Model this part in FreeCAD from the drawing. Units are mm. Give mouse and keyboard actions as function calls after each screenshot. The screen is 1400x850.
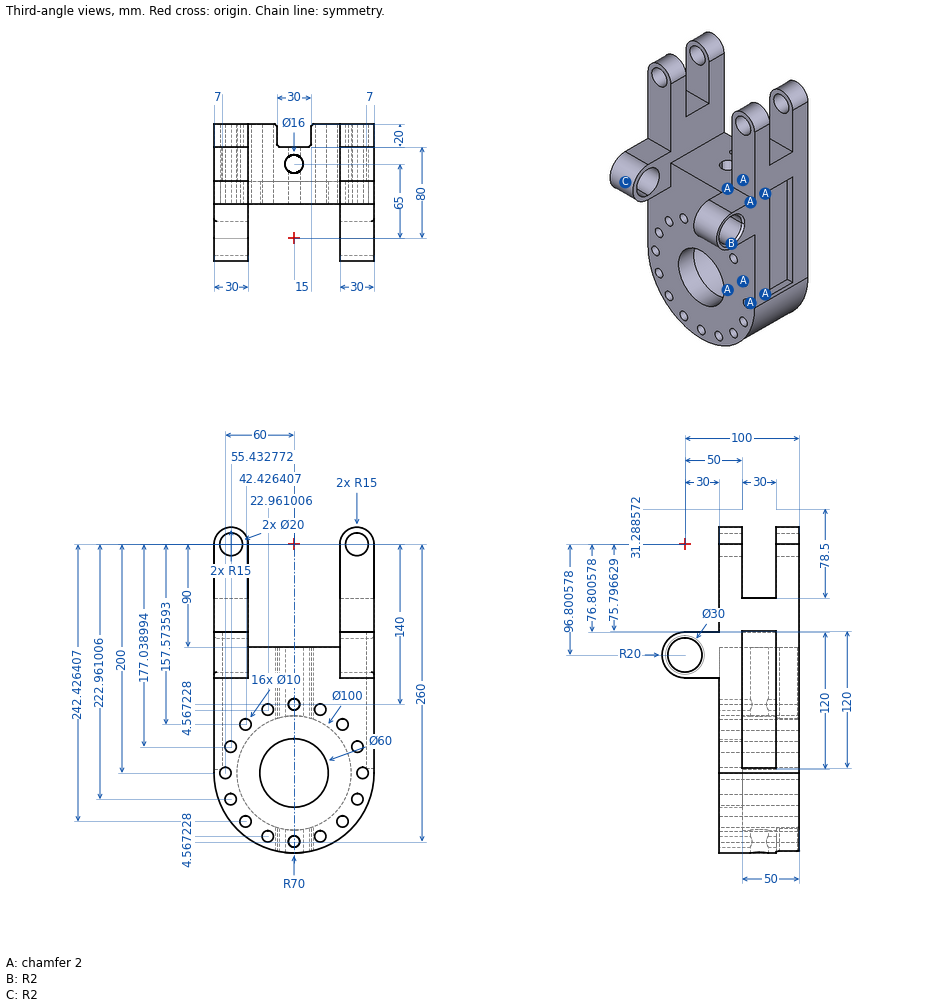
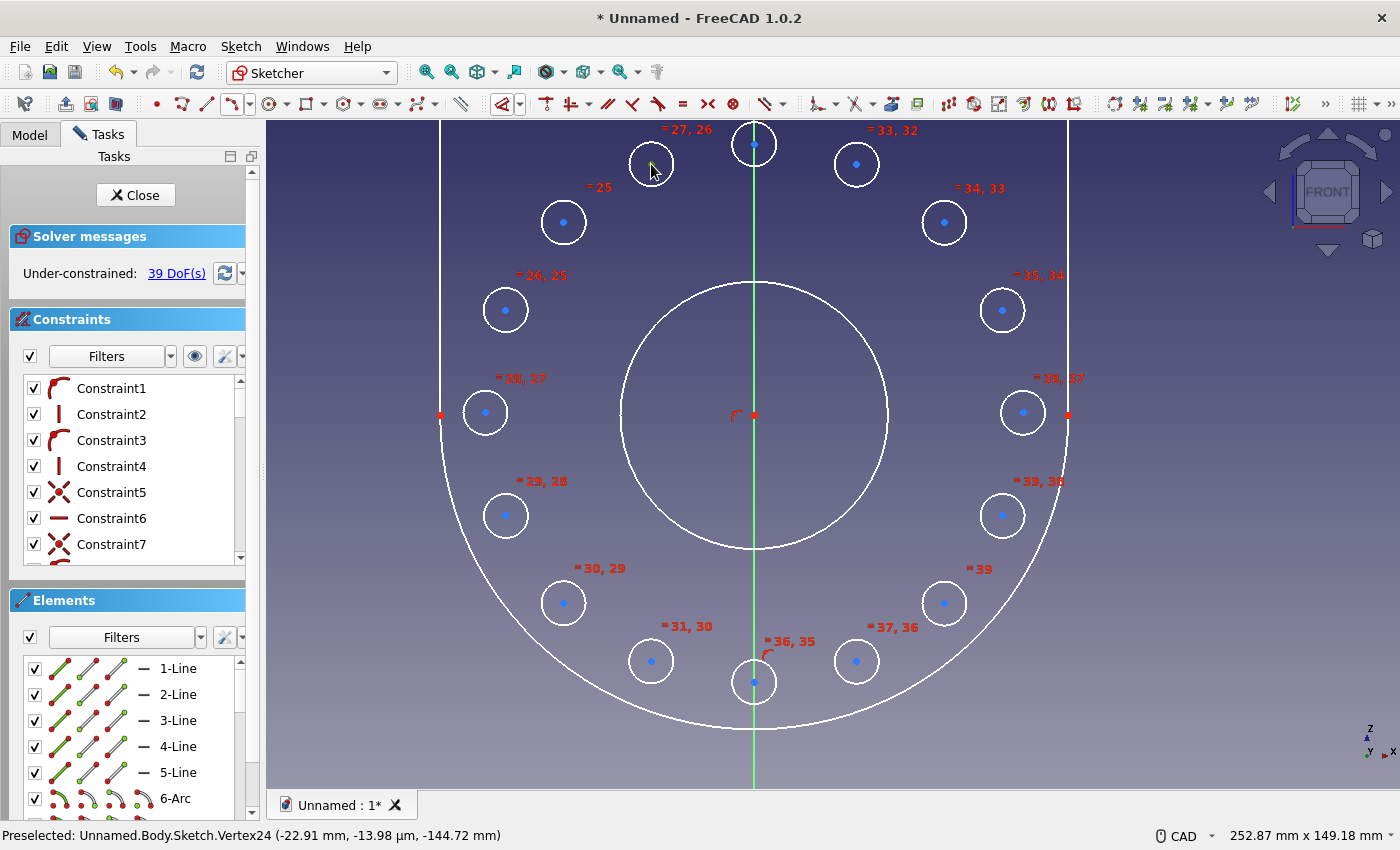
click(857, 165)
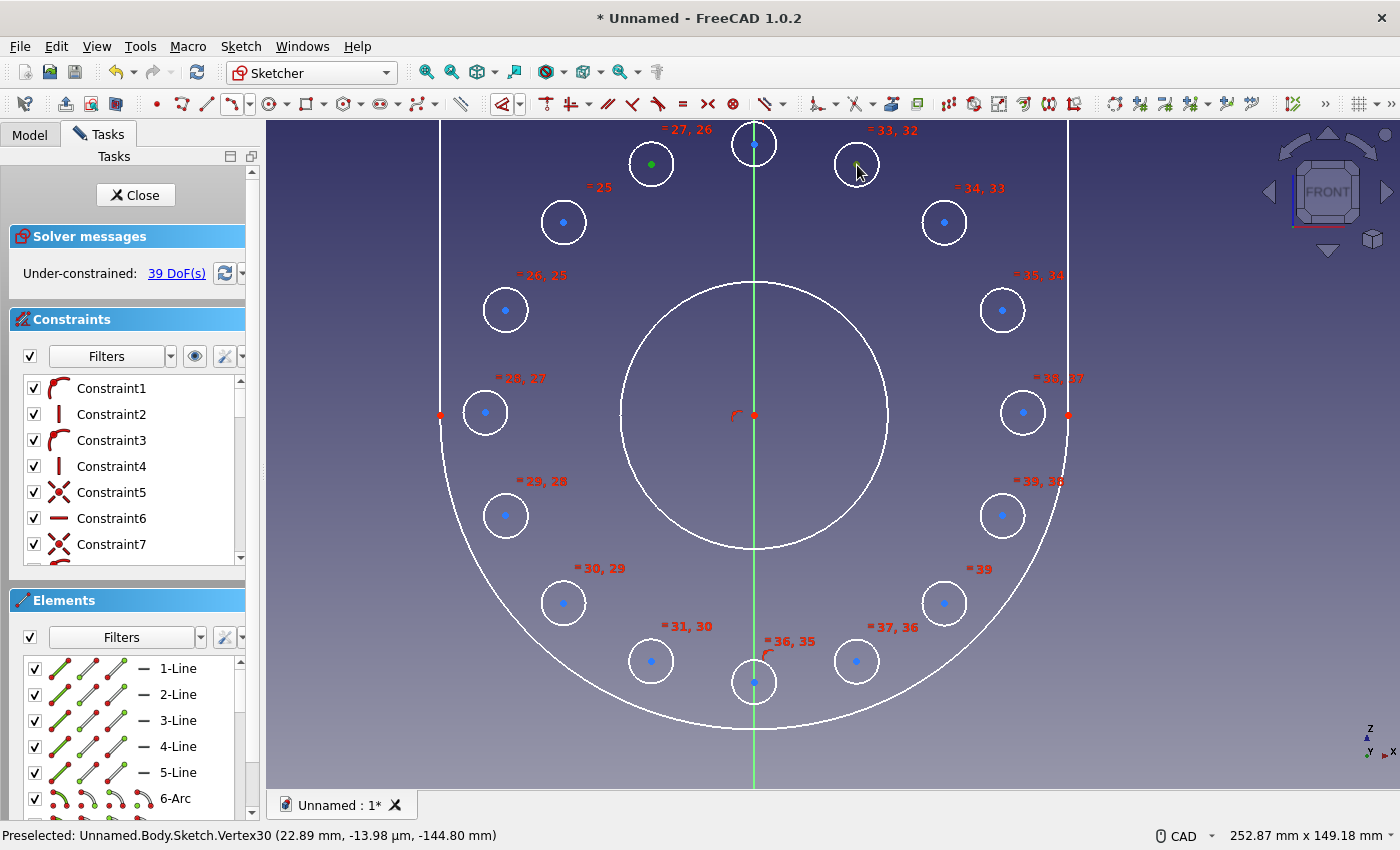
click(754, 630)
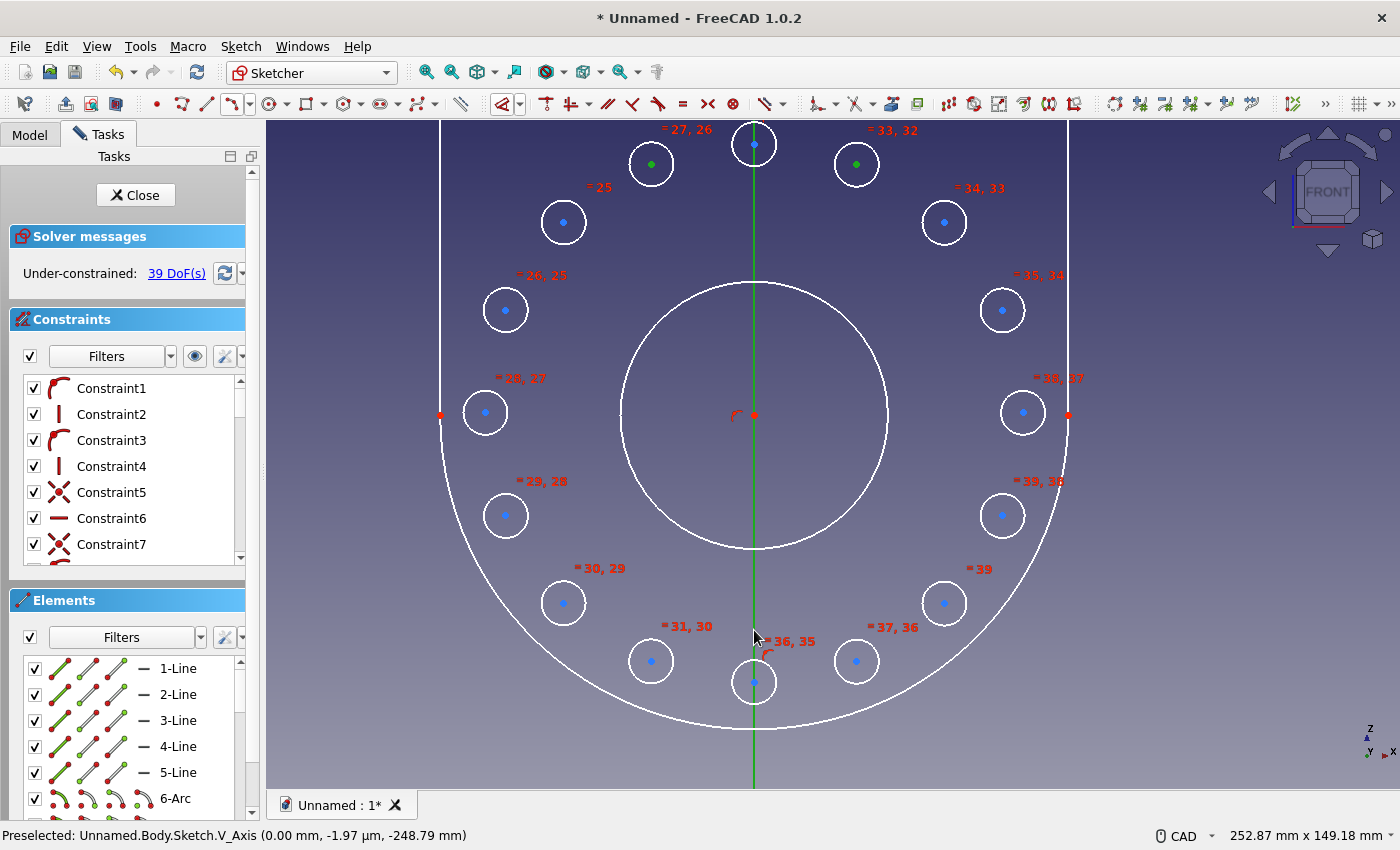
key(s)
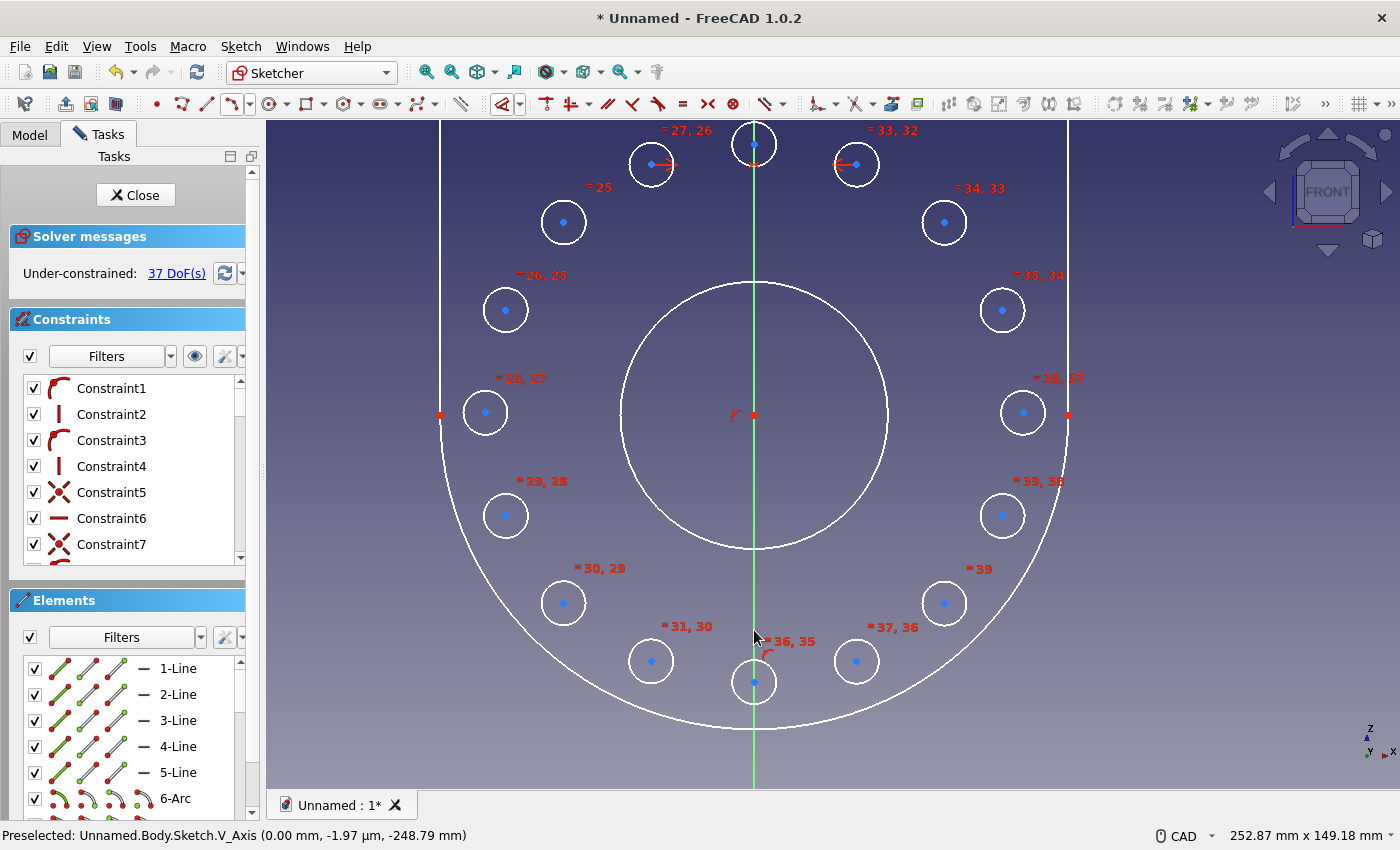
click(564, 222)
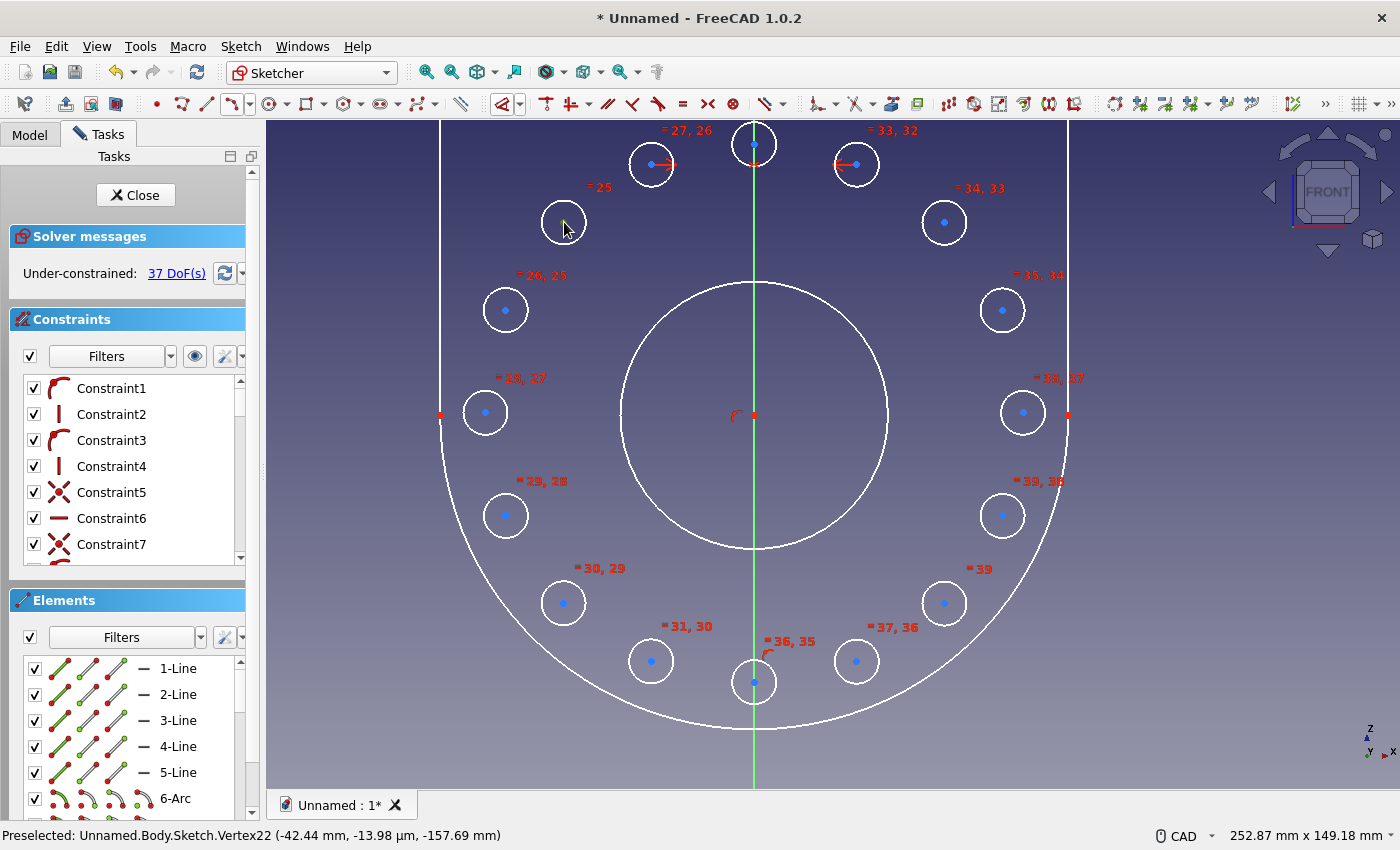
click(944, 223)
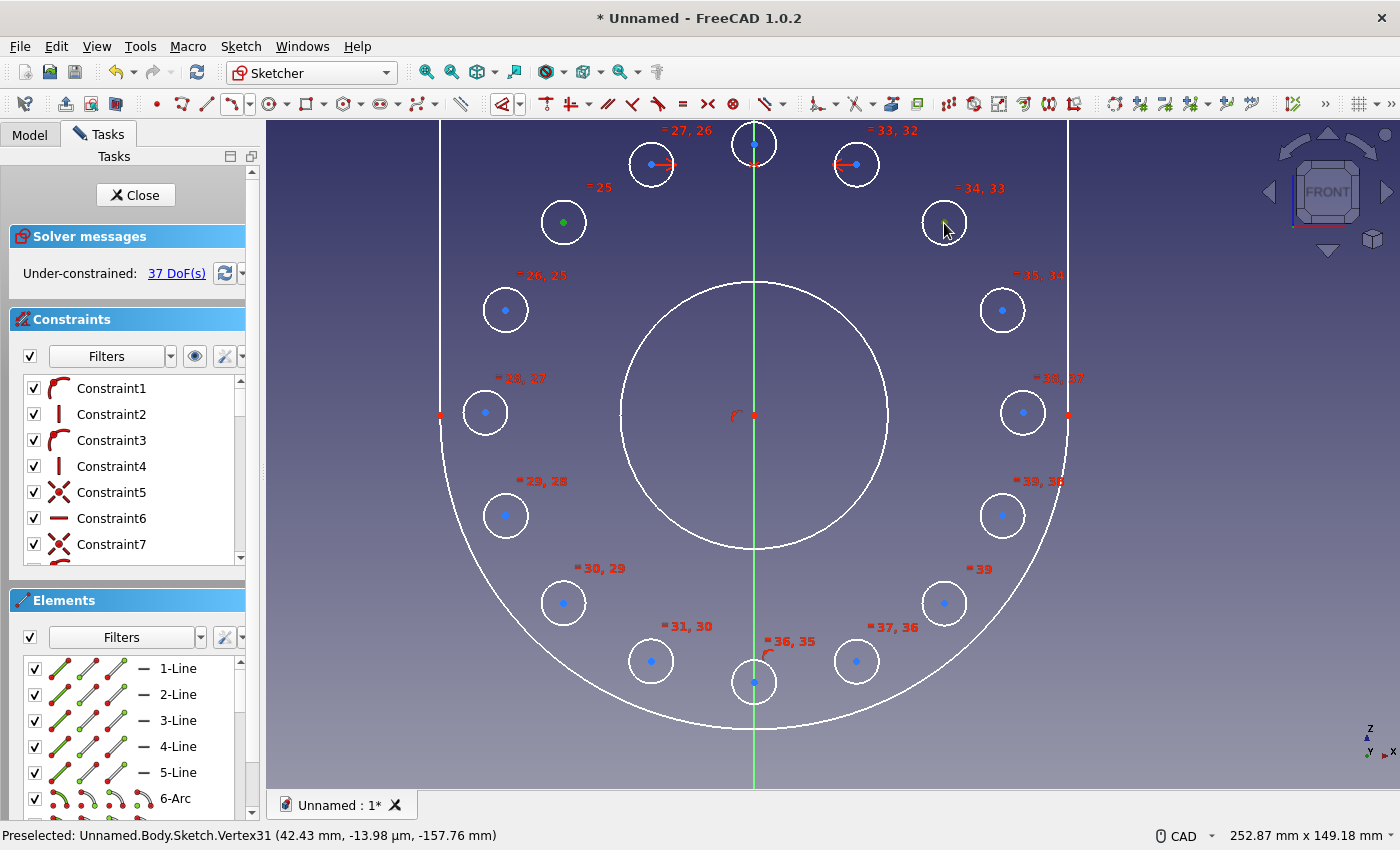
click(754, 630)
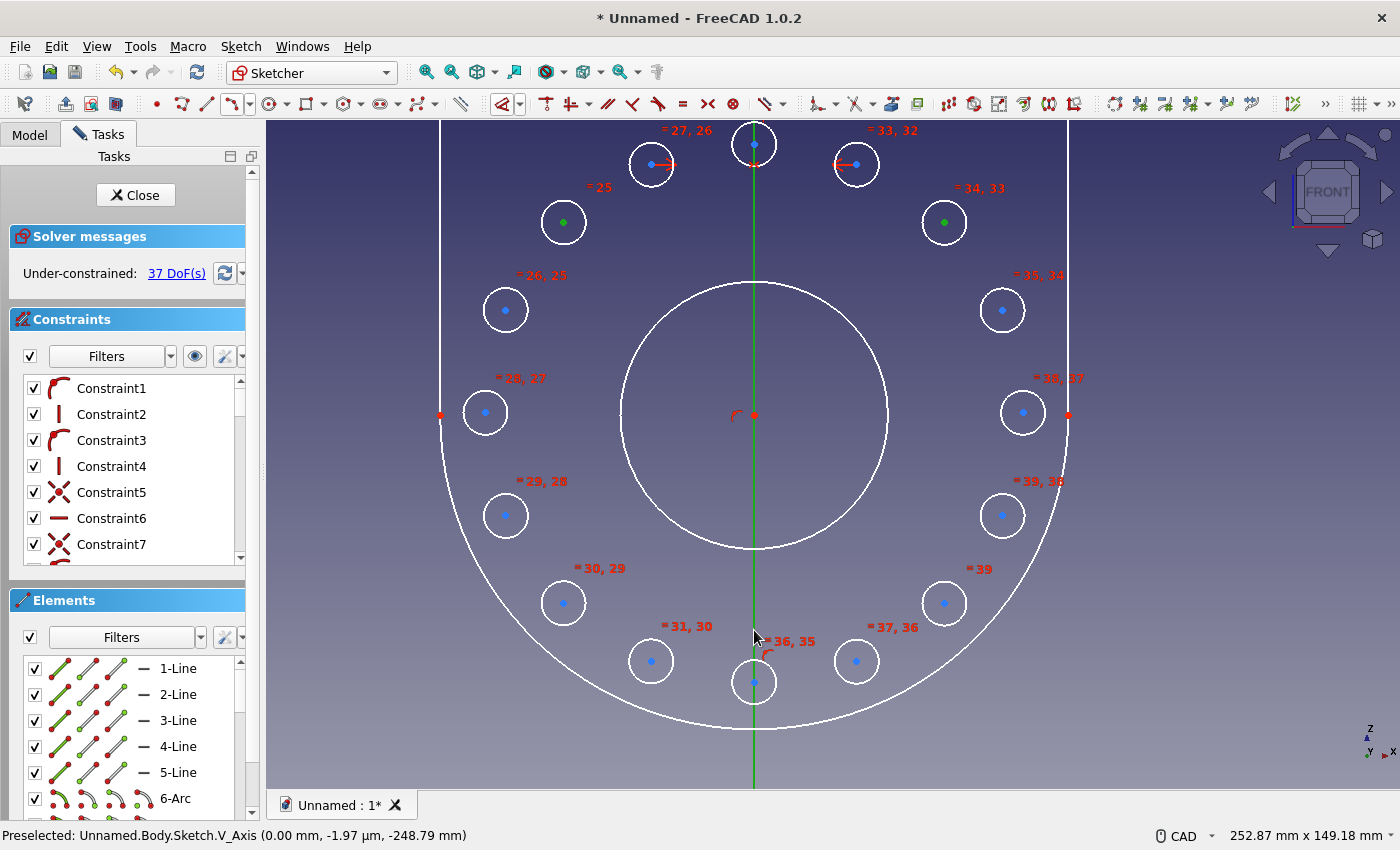
key(s)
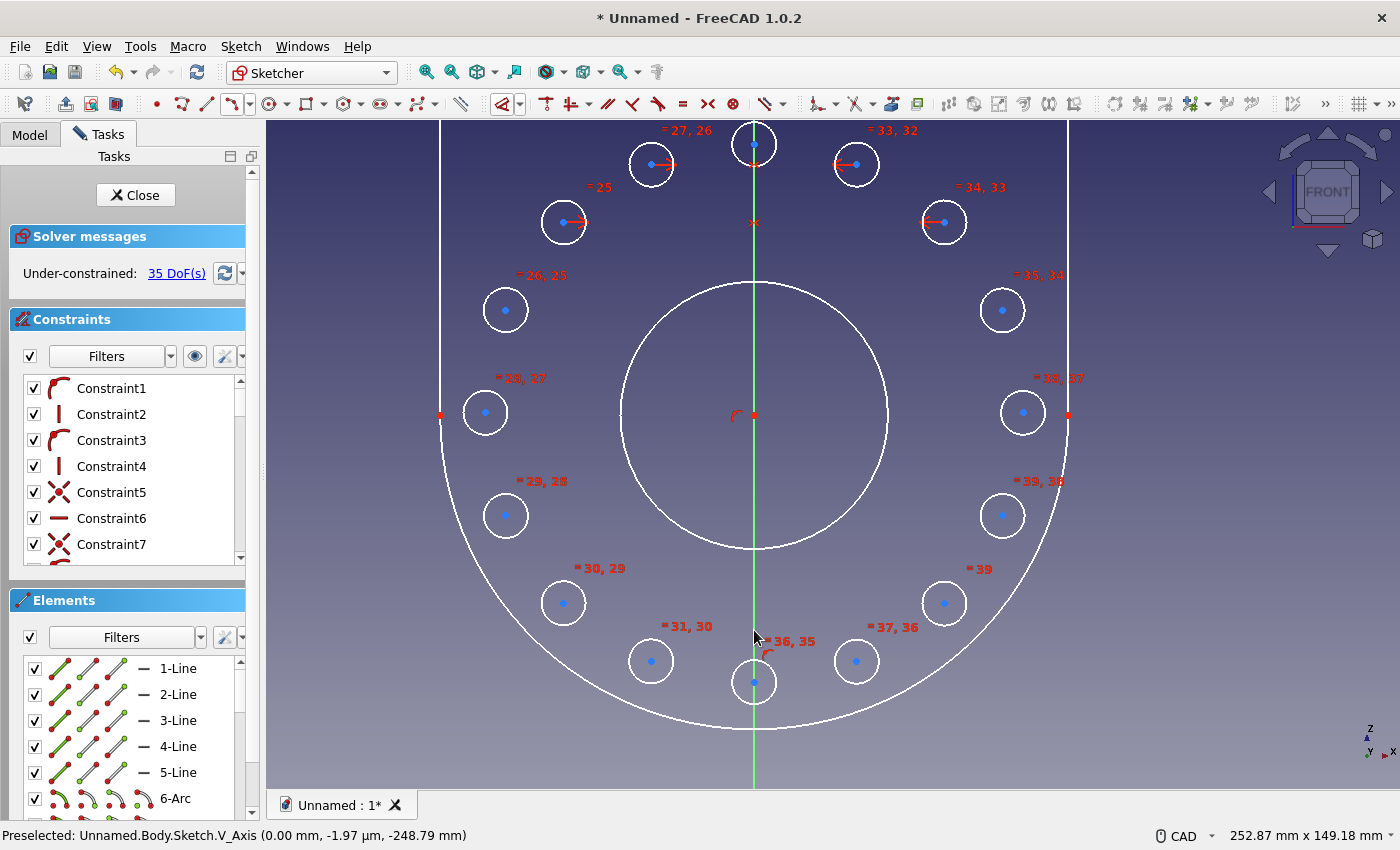
click(506, 310)